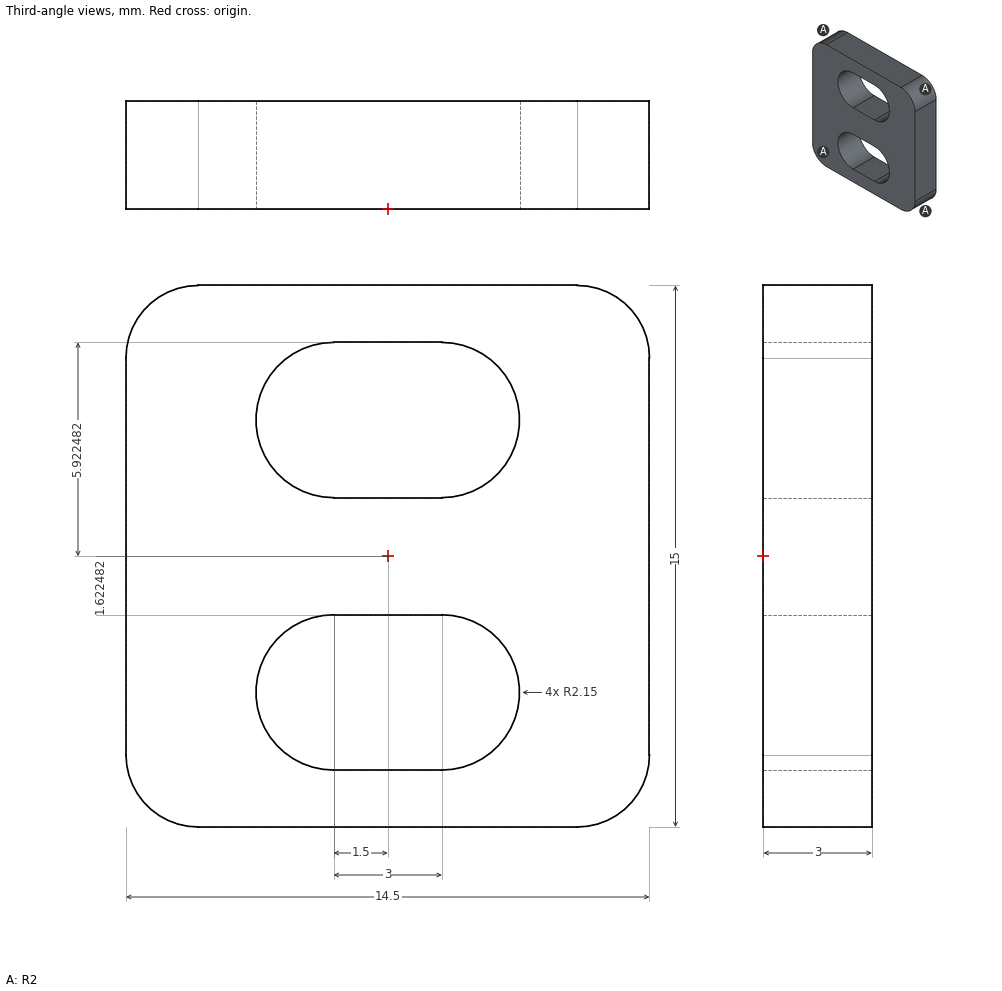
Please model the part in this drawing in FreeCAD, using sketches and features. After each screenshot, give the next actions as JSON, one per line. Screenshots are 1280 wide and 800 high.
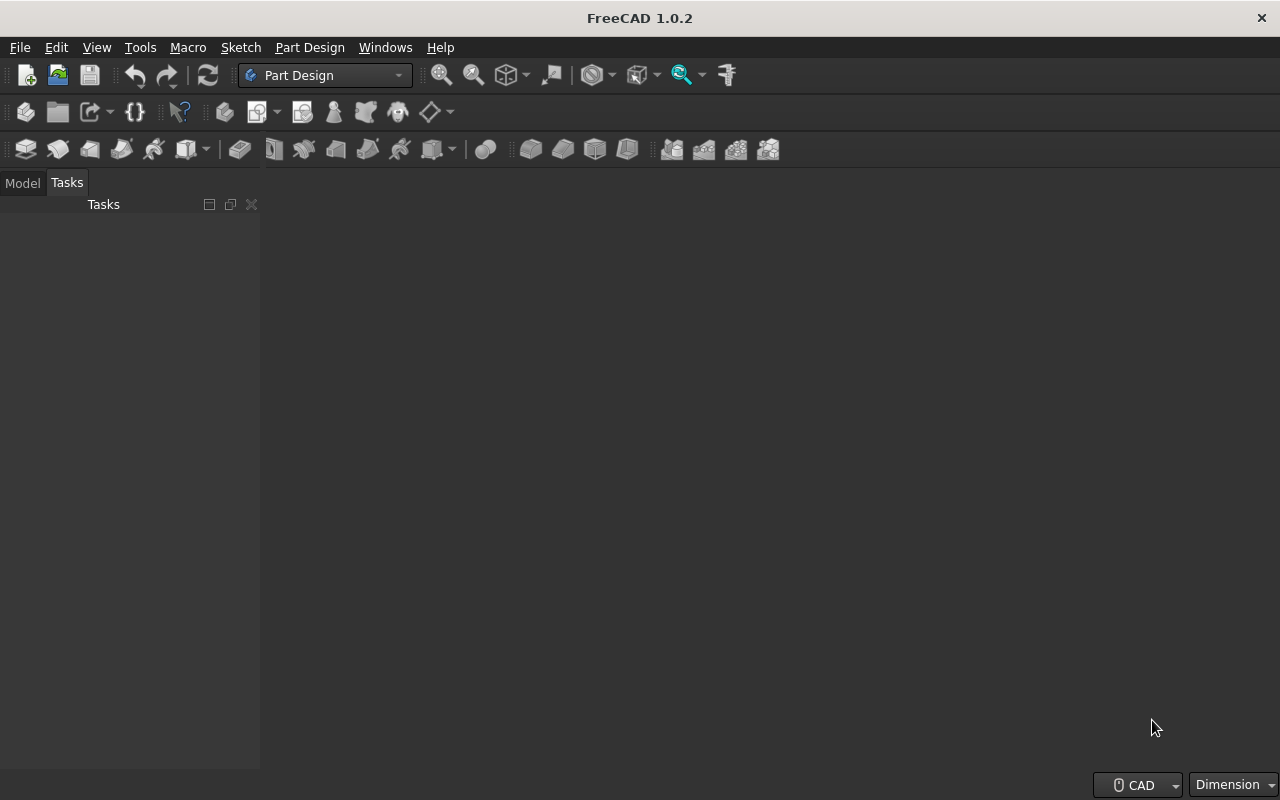
{"action": "left_click", "coordinate": [26, 76]}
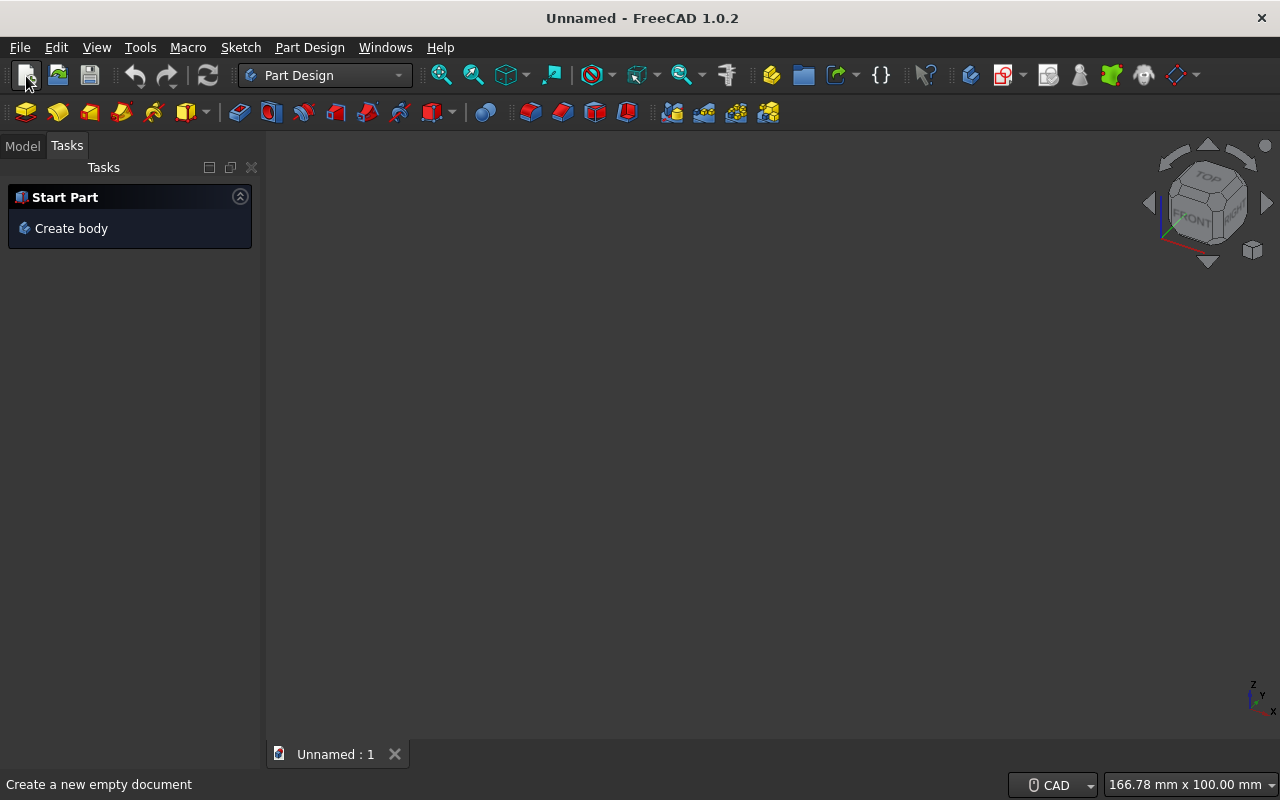
{"action": "left_click", "coordinate": [1004, 76]}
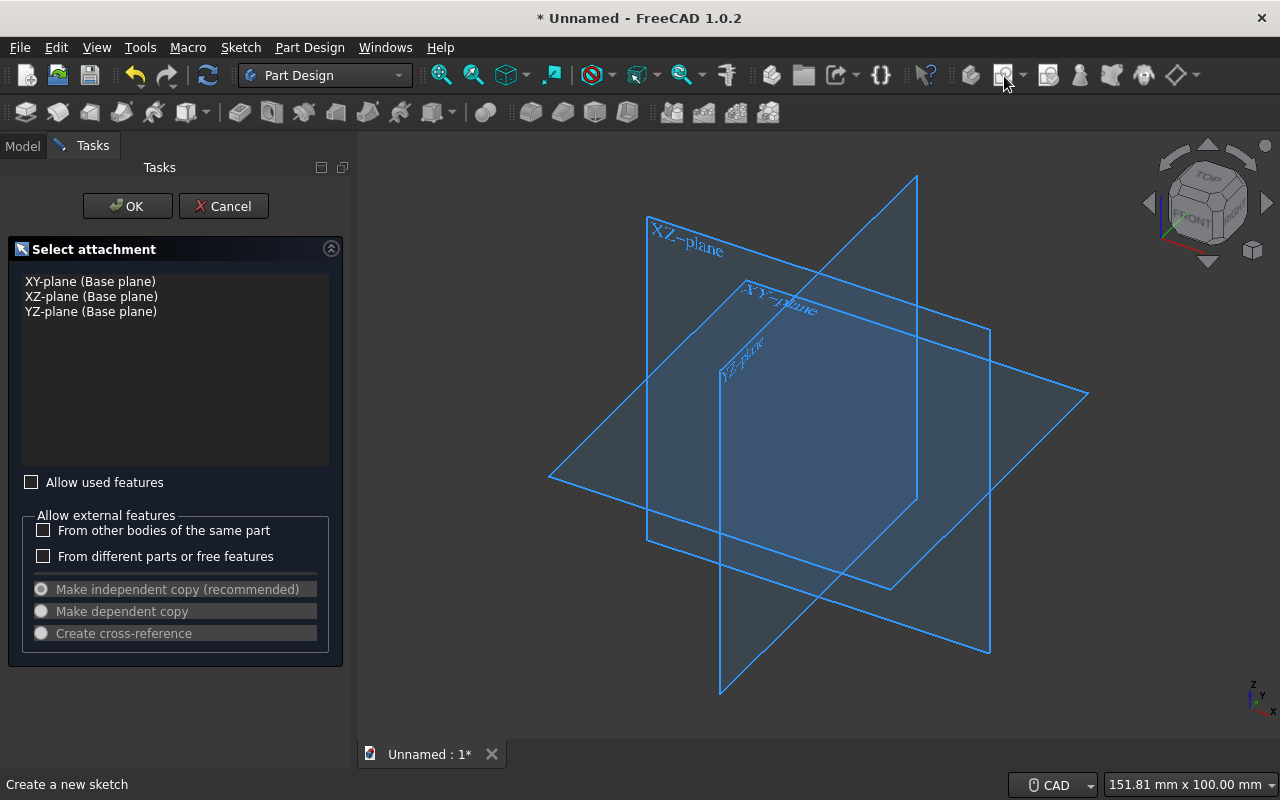
{"action": "left_click", "coordinate": [82, 296]}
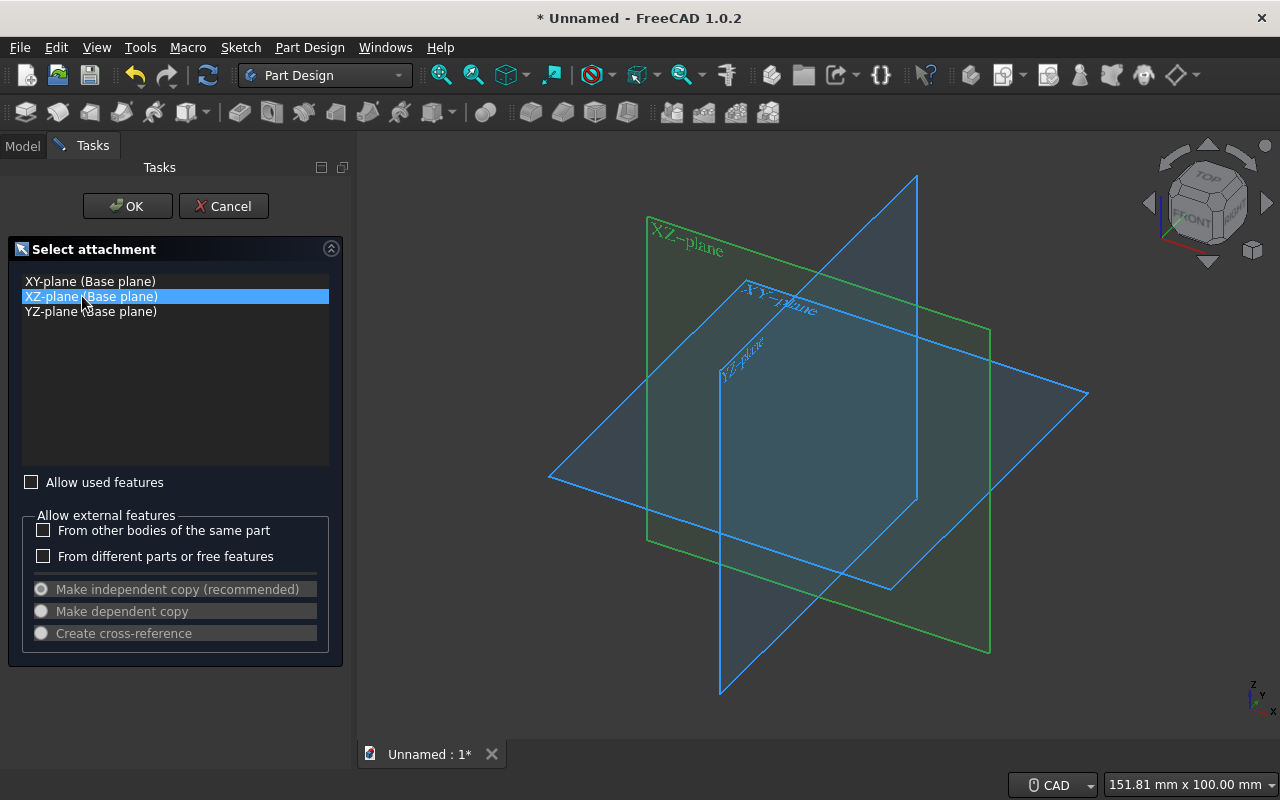
{"action": "left_click", "coordinate": [128, 206]}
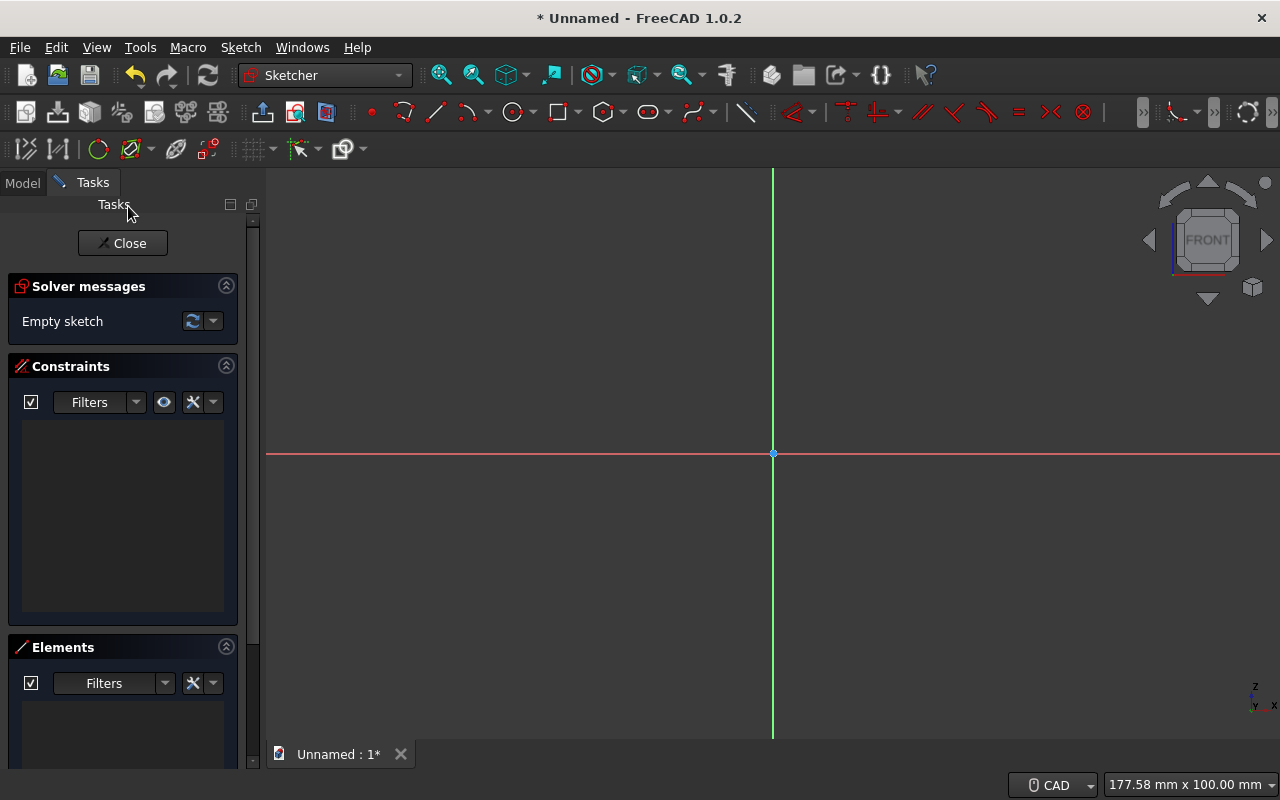
{"action": "scroll", "coordinate": [795, 454], "scroll_direction": "up", "scroll_amount": 7}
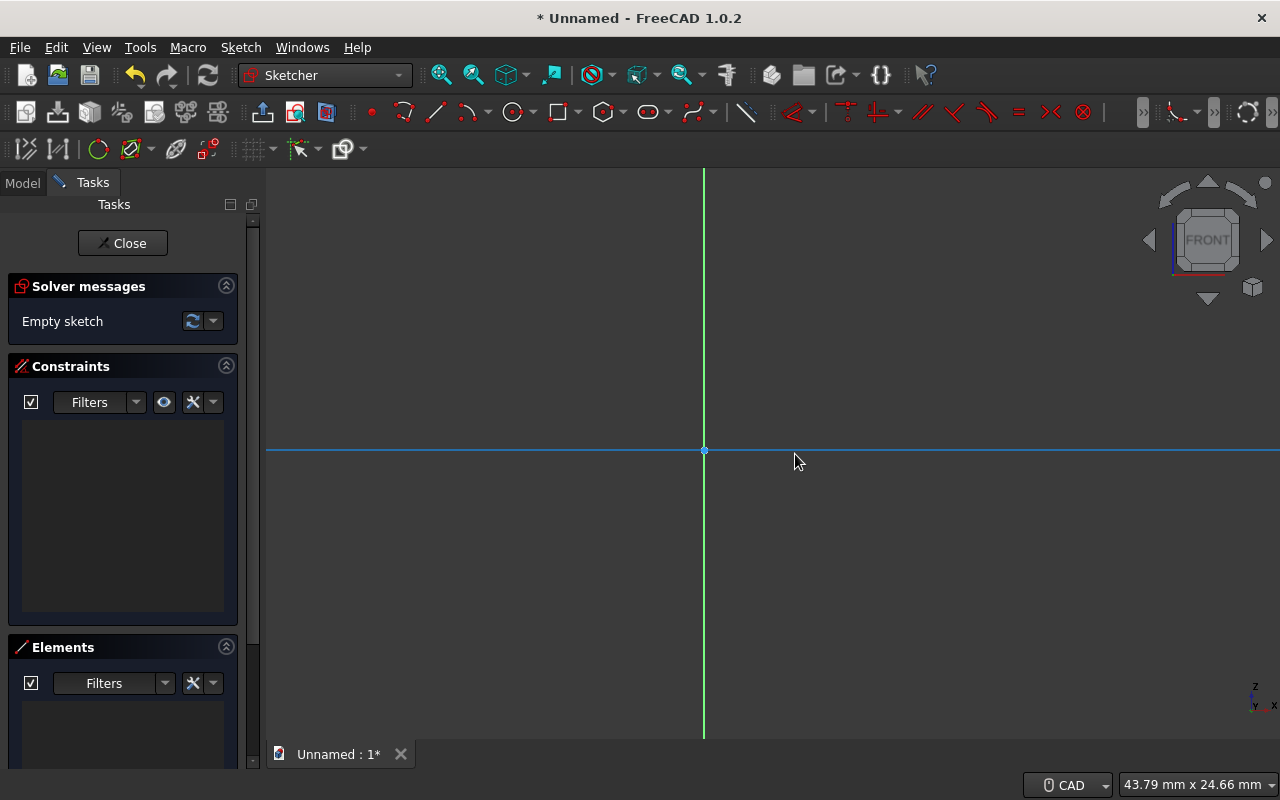
{"action": "key", "text": "g v"}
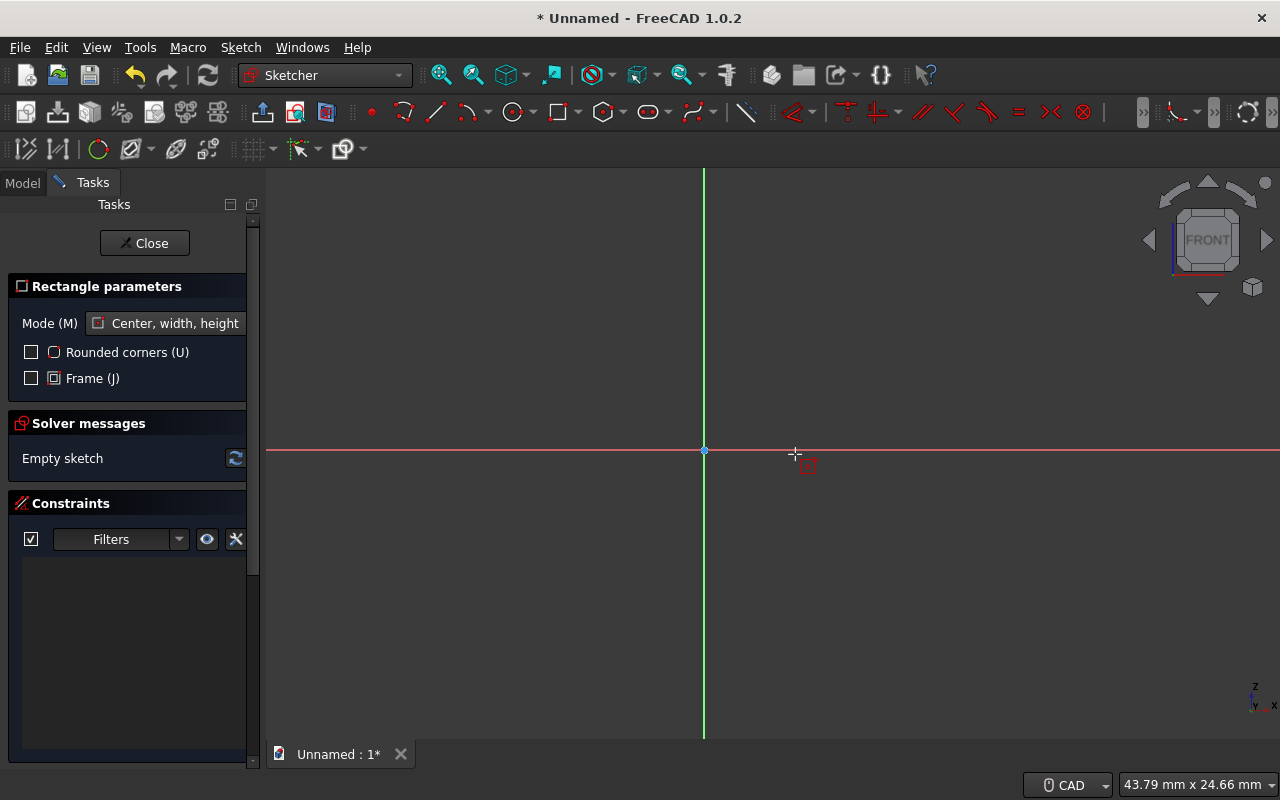
{"action": "left_click", "coordinate": [704, 450]}
{"action": "mouse_move", "coordinate": [872, 277]}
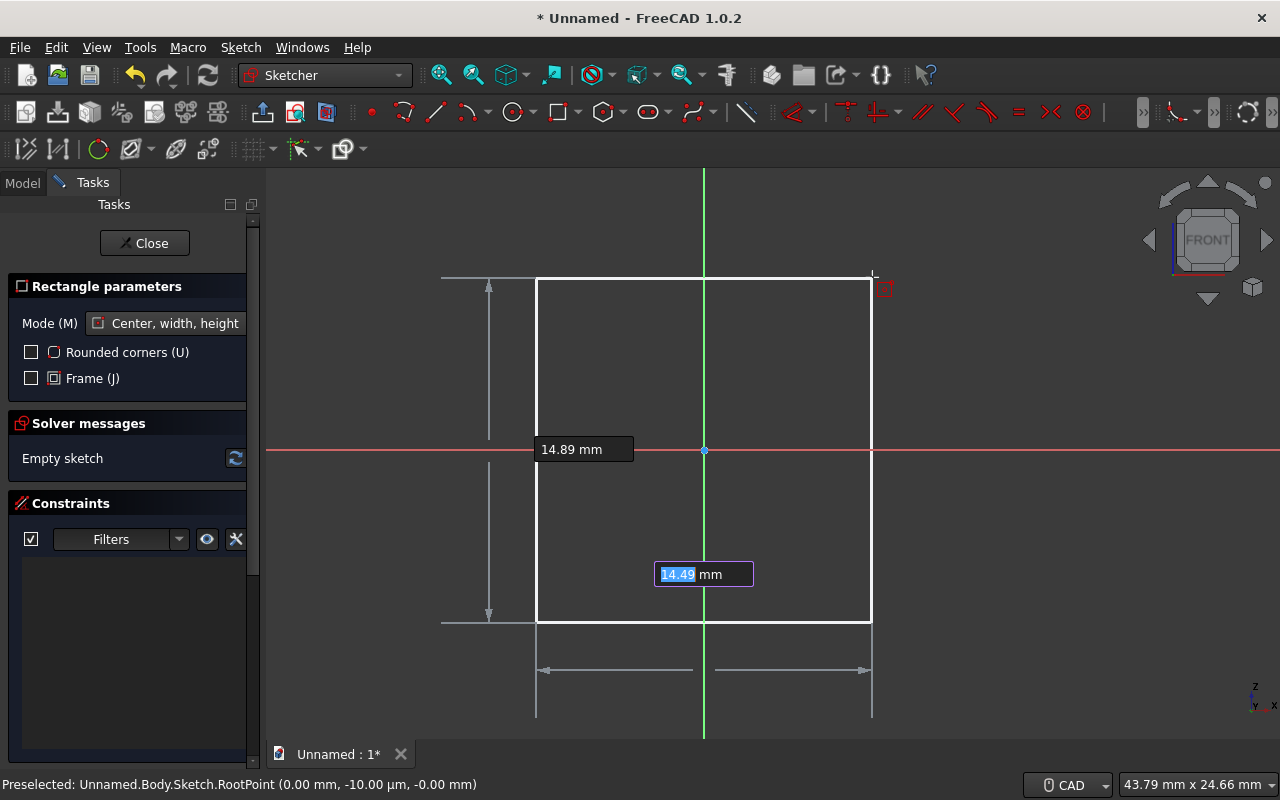
{"action": "type", "text": "14.5"}
{"action": "key", "text": "Tab"}
{"action": "type", "text": "15"}
{"action": "key", "text": "Return"}
{"action": "key", "text": "Escape"}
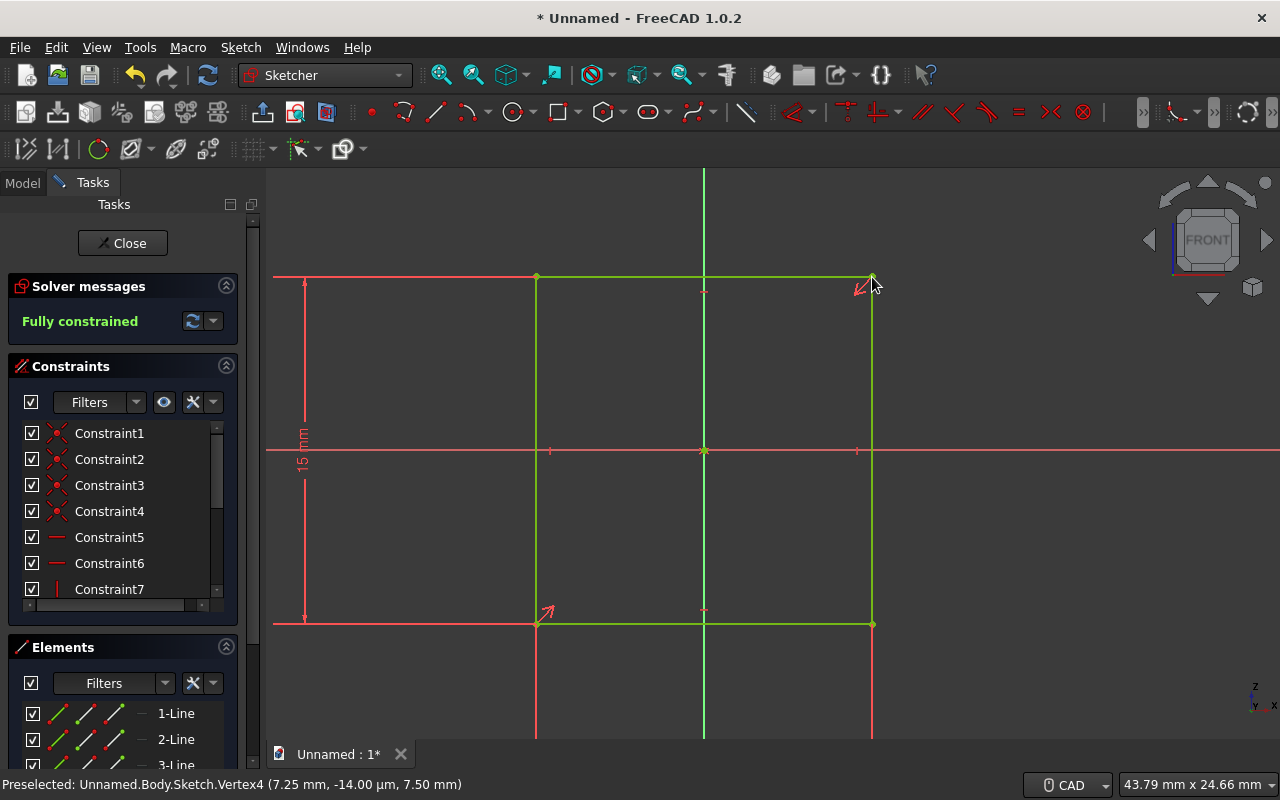
{"action": "left_click", "coordinate": [123, 243]}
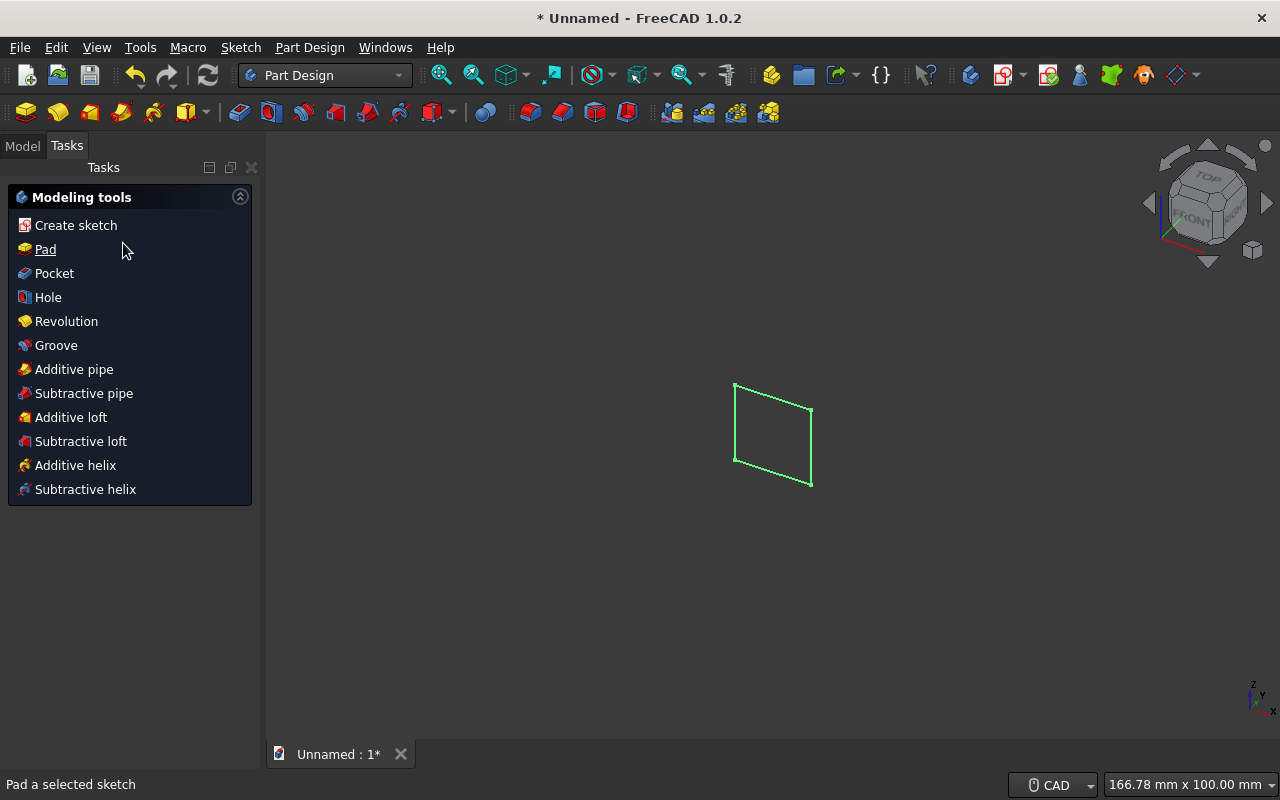
{"action": "left_click", "coordinate": [26, 112]}